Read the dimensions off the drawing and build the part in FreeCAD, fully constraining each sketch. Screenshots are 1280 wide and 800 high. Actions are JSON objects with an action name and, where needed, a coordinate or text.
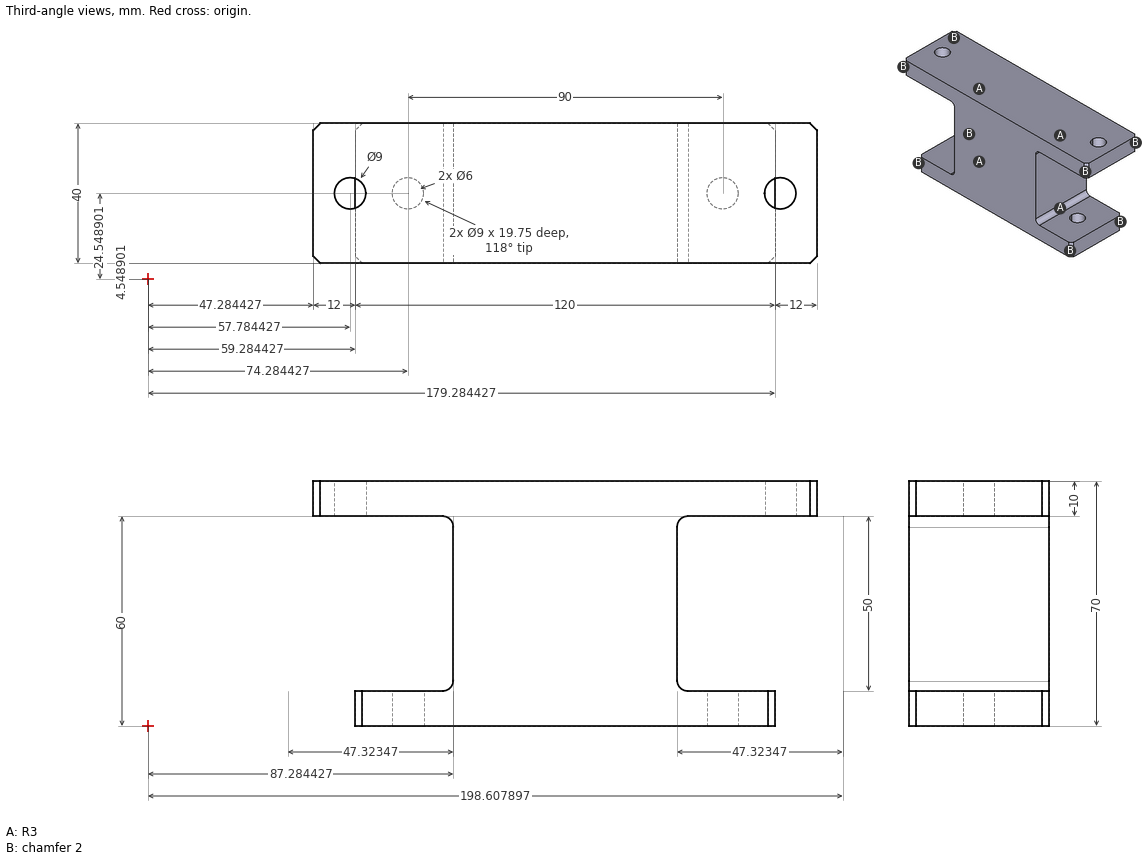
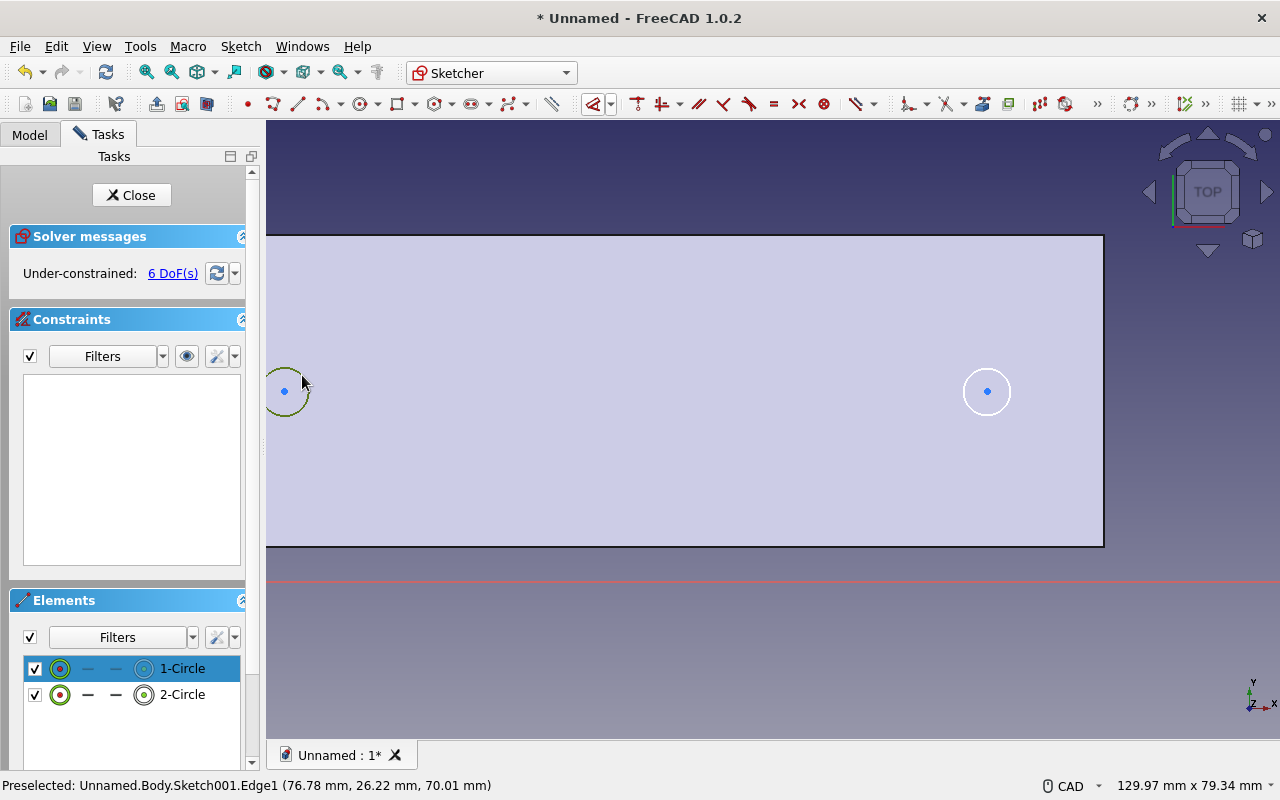
{"action": "left_click", "coordinate": [1003, 375]}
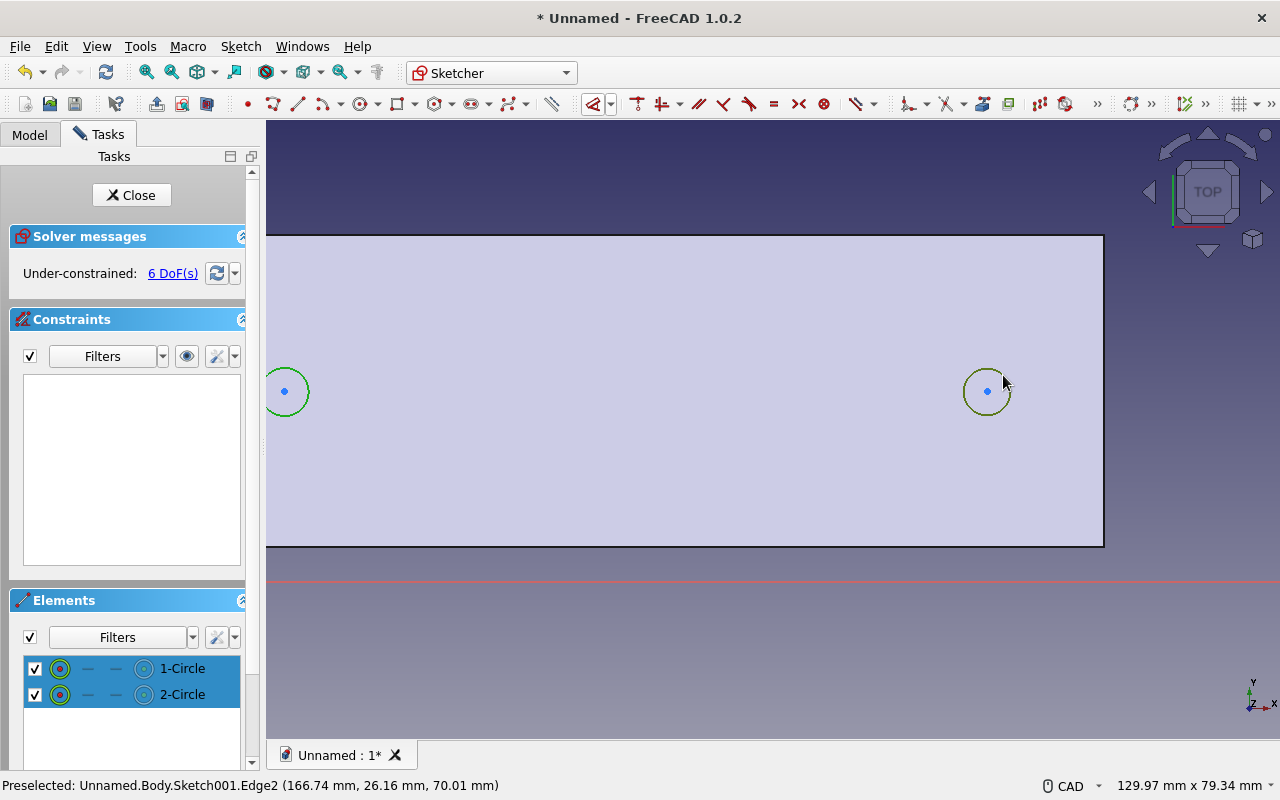
{"action": "key", "text": "e"}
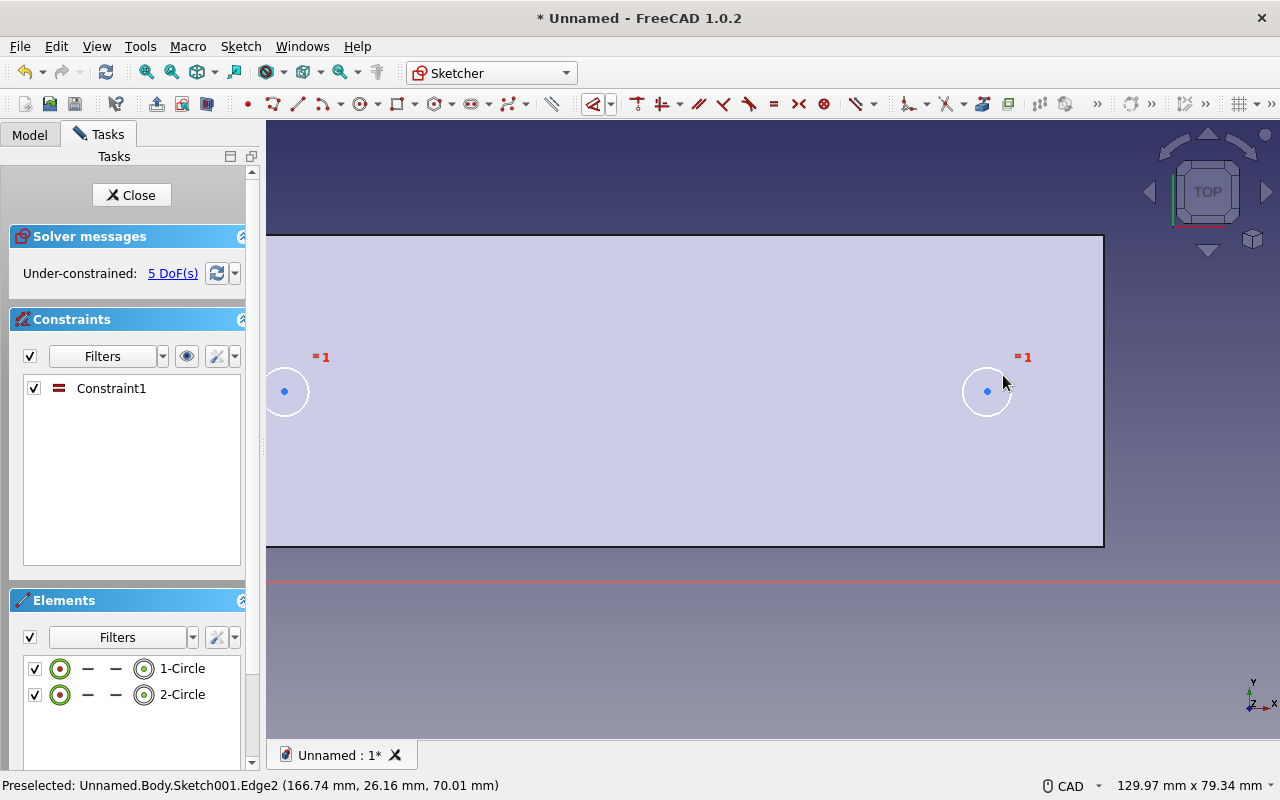
{"action": "scroll", "coordinate": [988, 392], "scroll_direction": "down", "scroll_amount": 4}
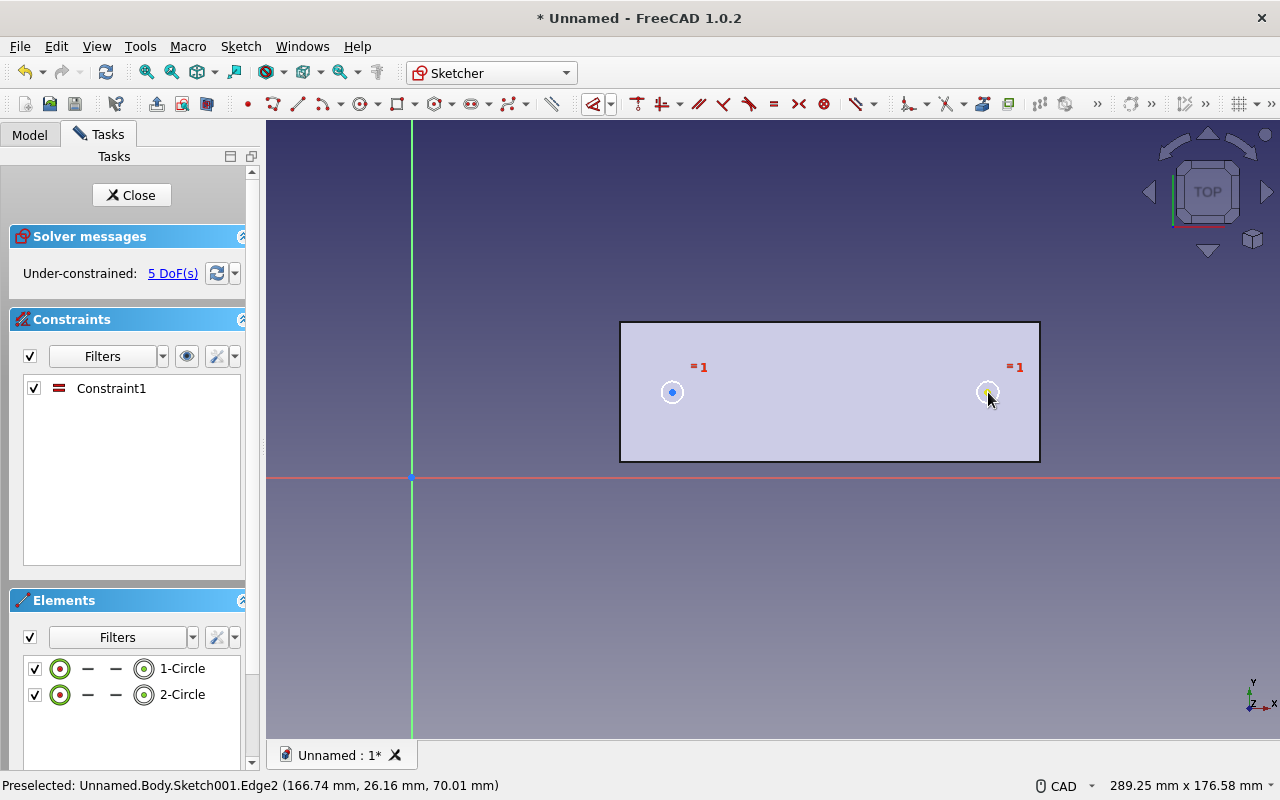
{"action": "left_click", "coordinate": [672, 392]}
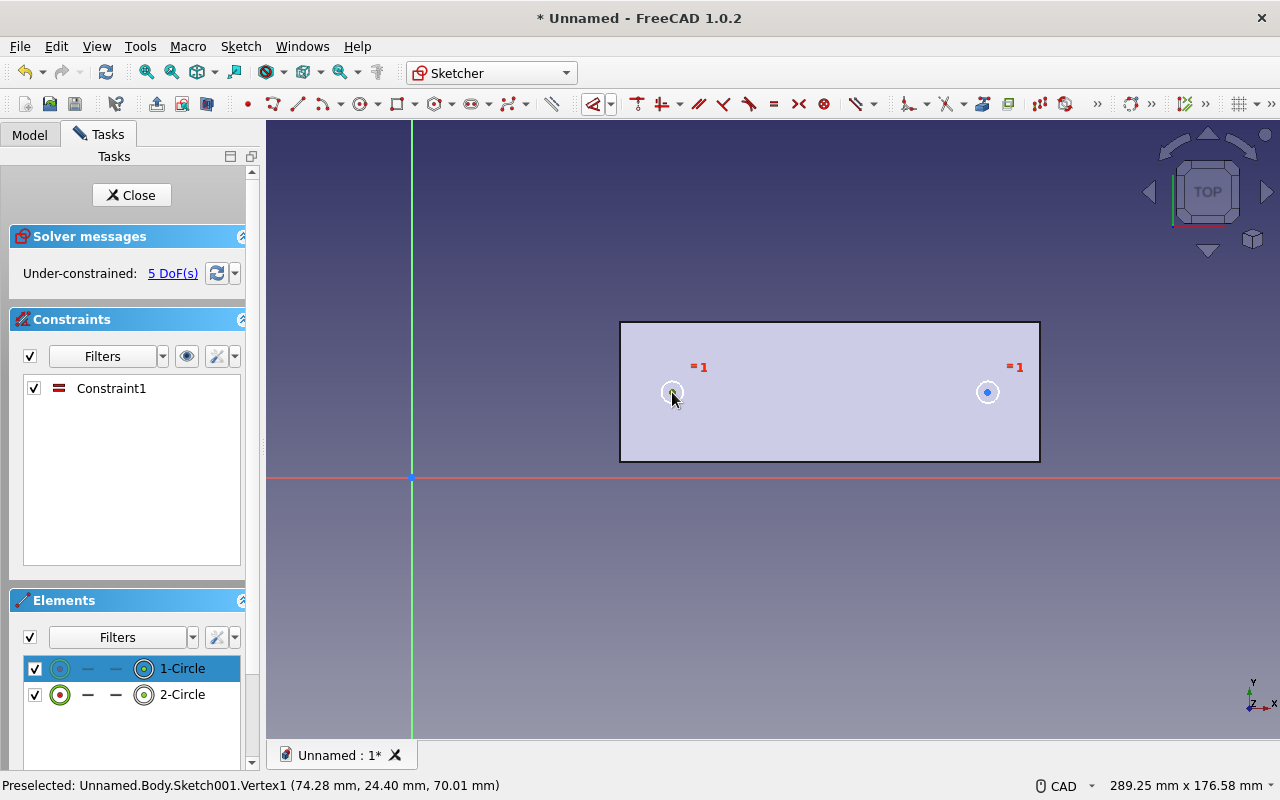
{"action": "left_click", "coordinate": [988, 392]}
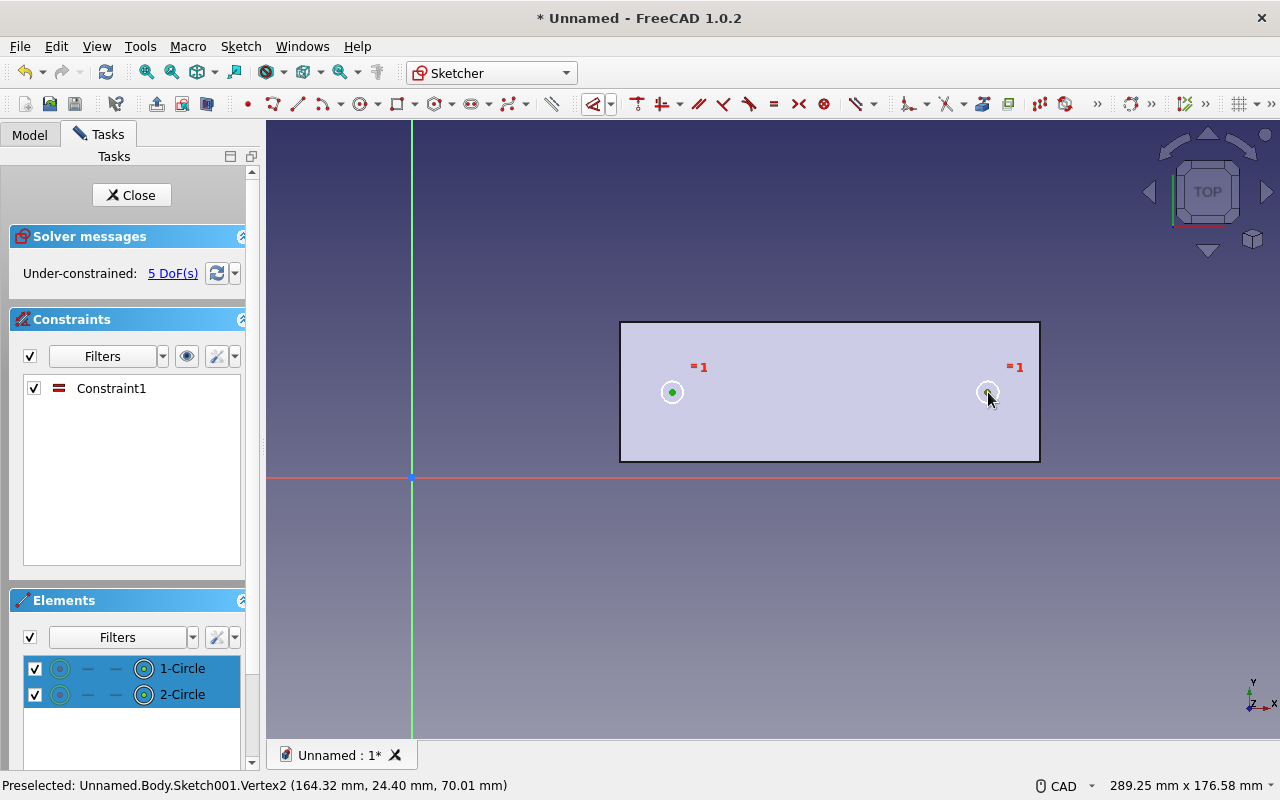
{"action": "key", "text": "h"}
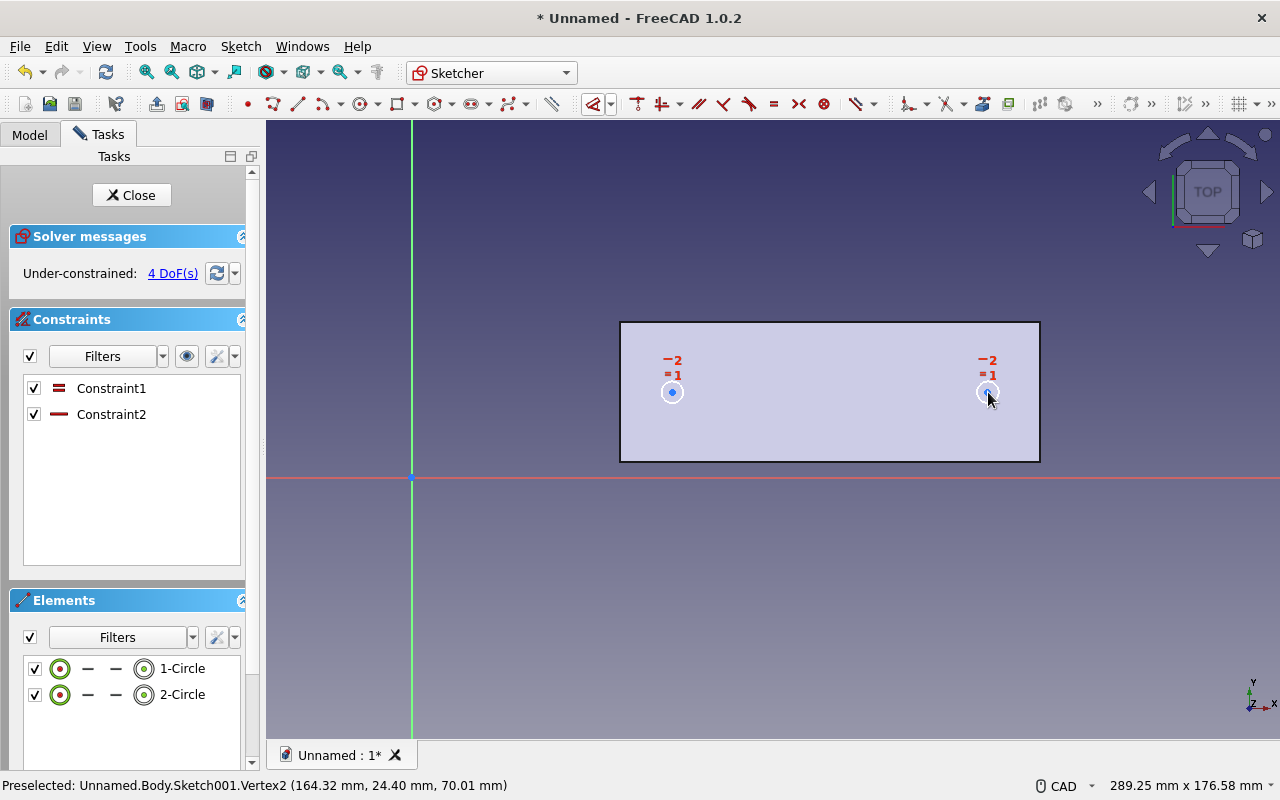
{"action": "scroll", "coordinate": [680, 385], "scroll_direction": "up", "scroll_amount": 4}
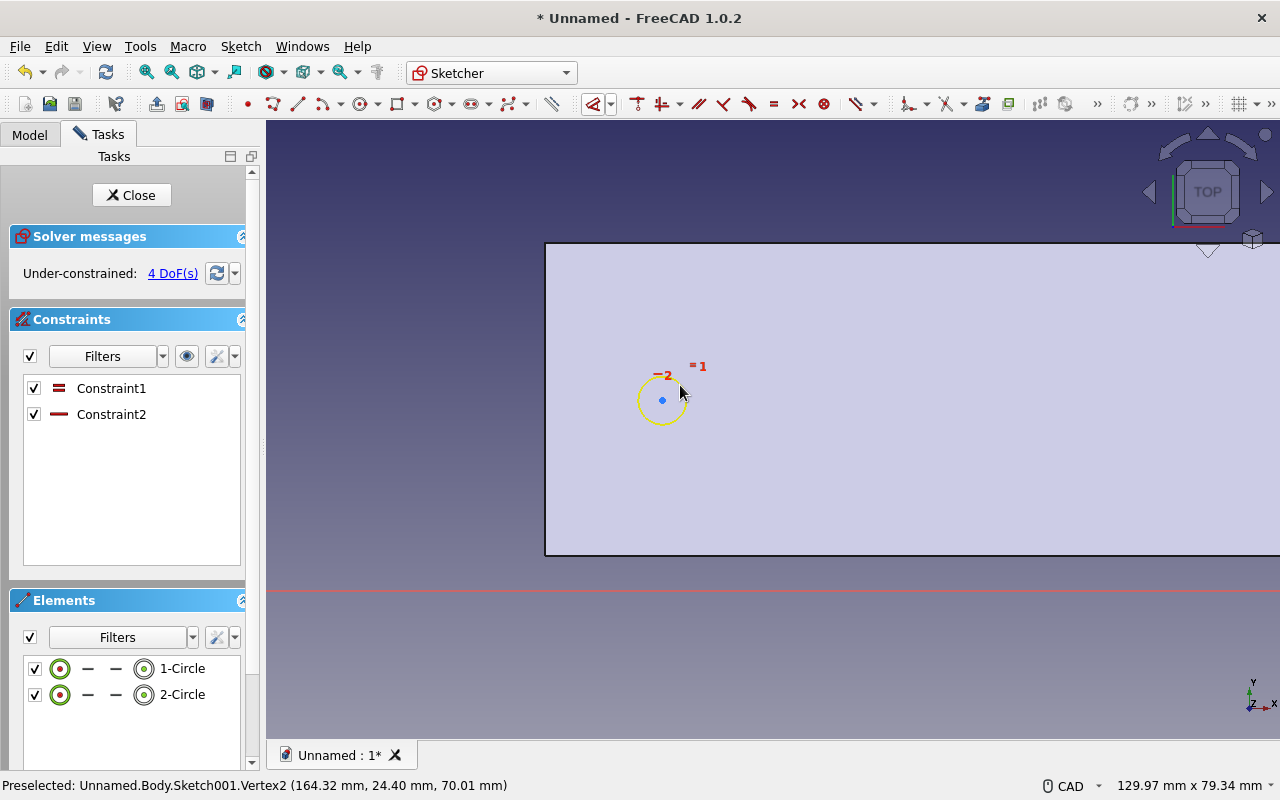
{"action": "left_click", "coordinate": [679, 384]}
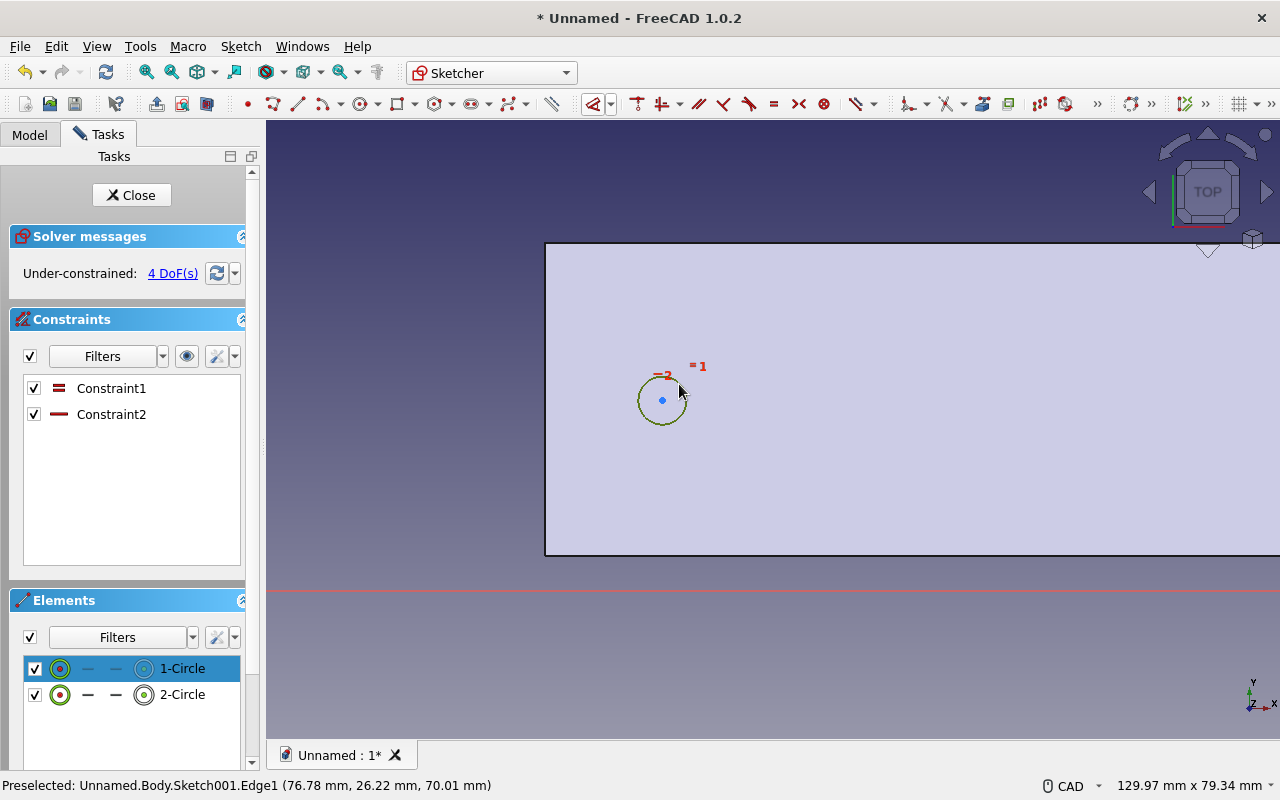
{"action": "key", "text": "k o"}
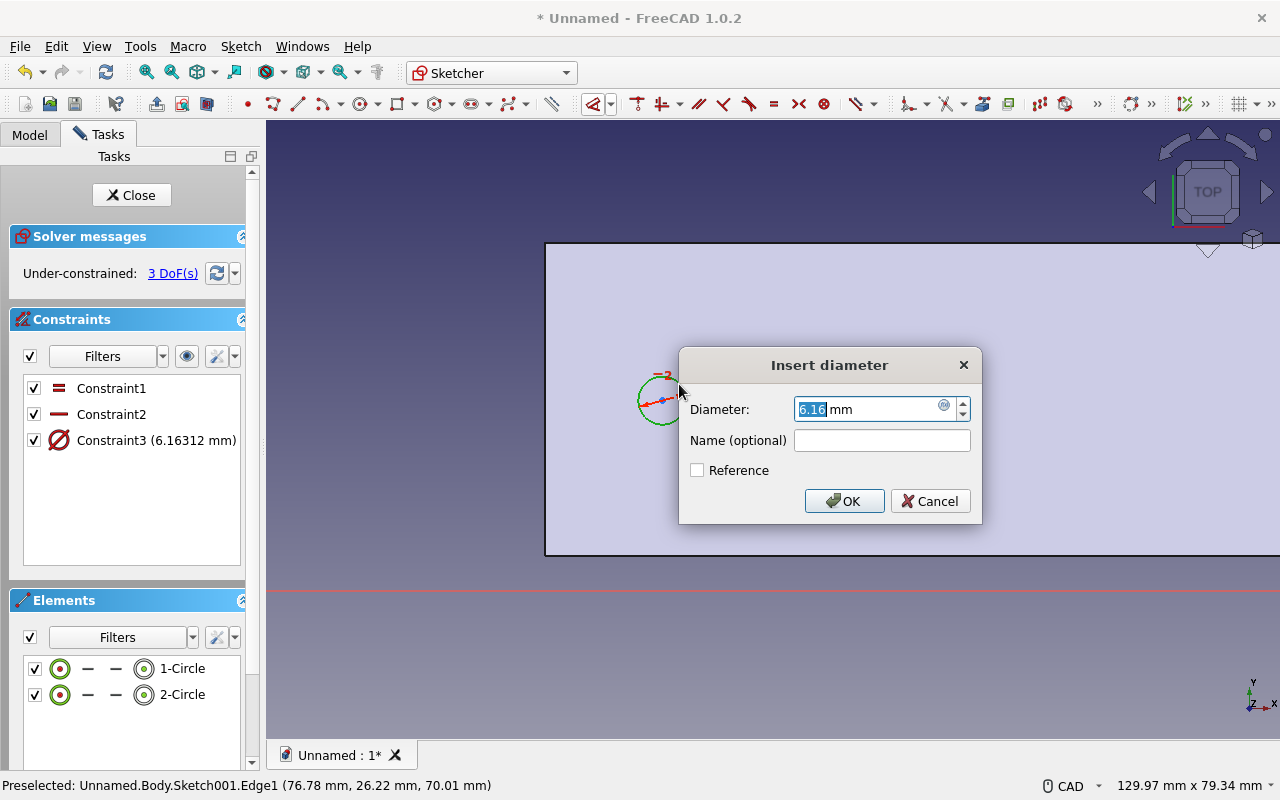
{"action": "type", "text": "6"}
{"action": "key", "text": "Return"}